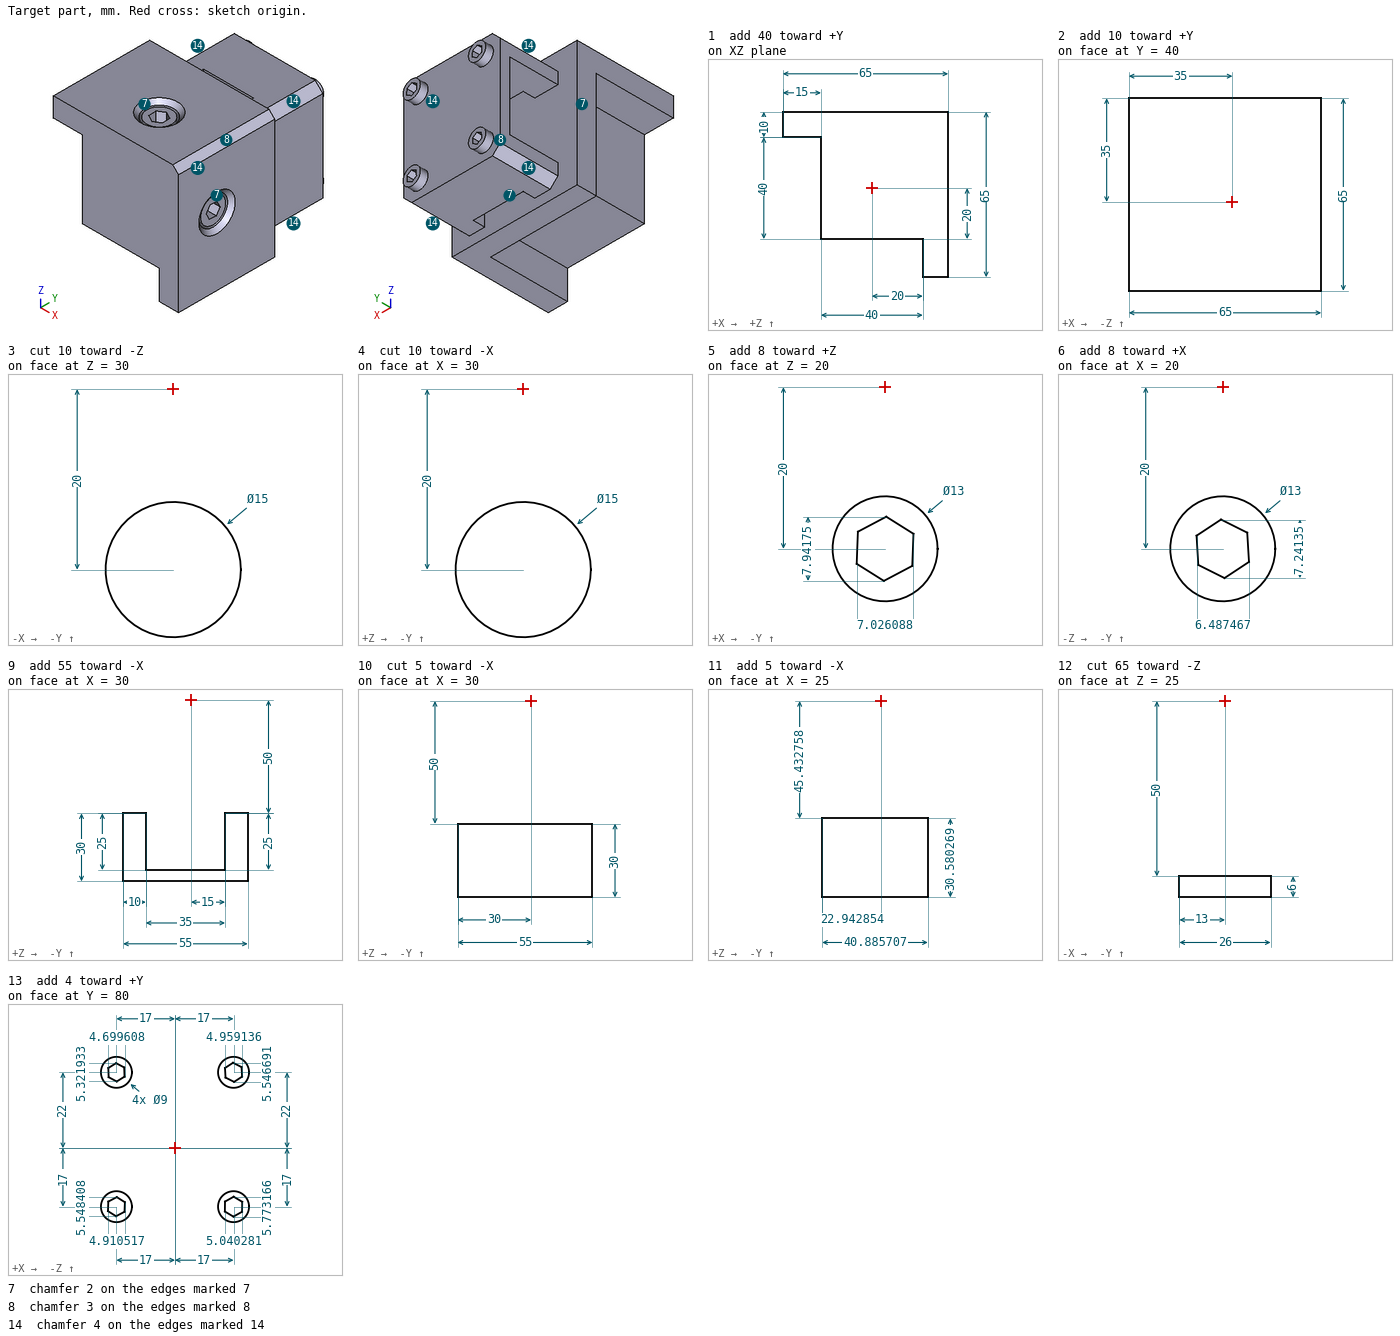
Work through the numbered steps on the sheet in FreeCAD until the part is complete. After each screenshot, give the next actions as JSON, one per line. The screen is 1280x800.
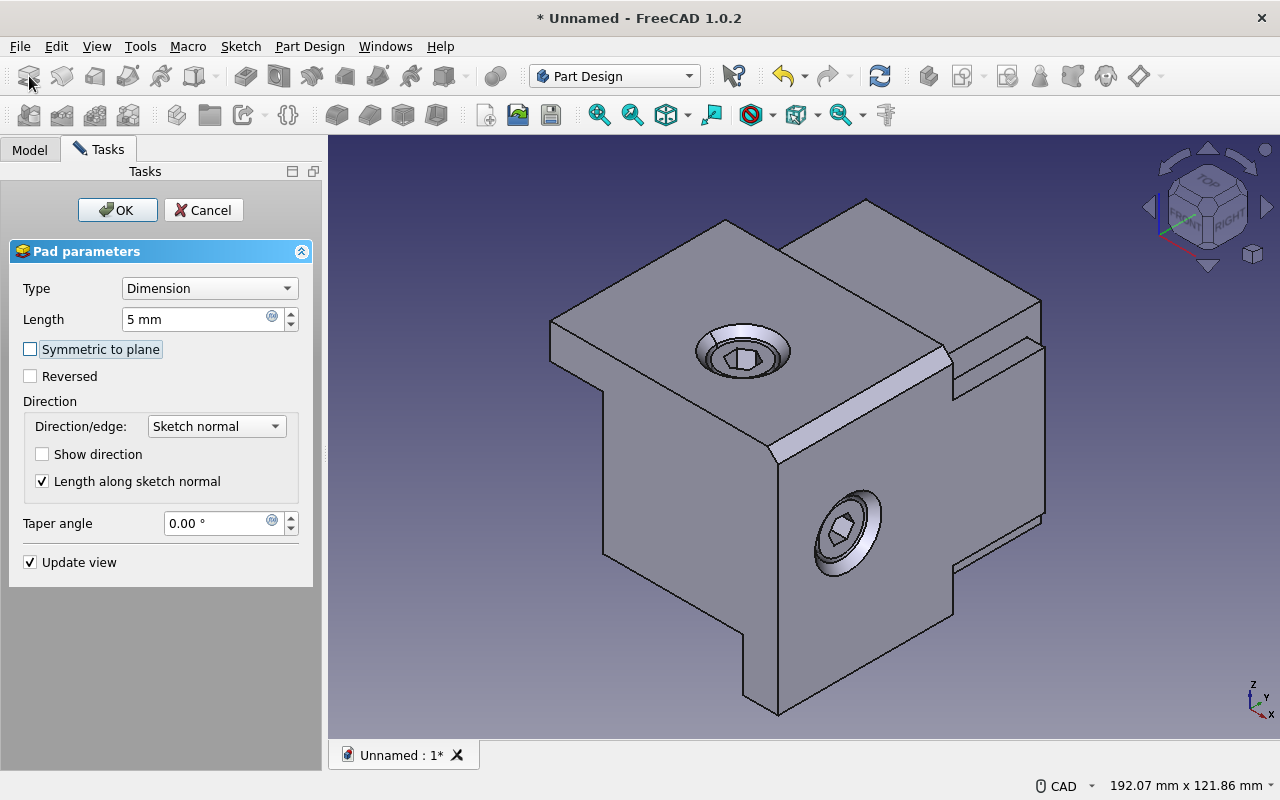
{"action": "left_click", "coordinate": [31, 376]}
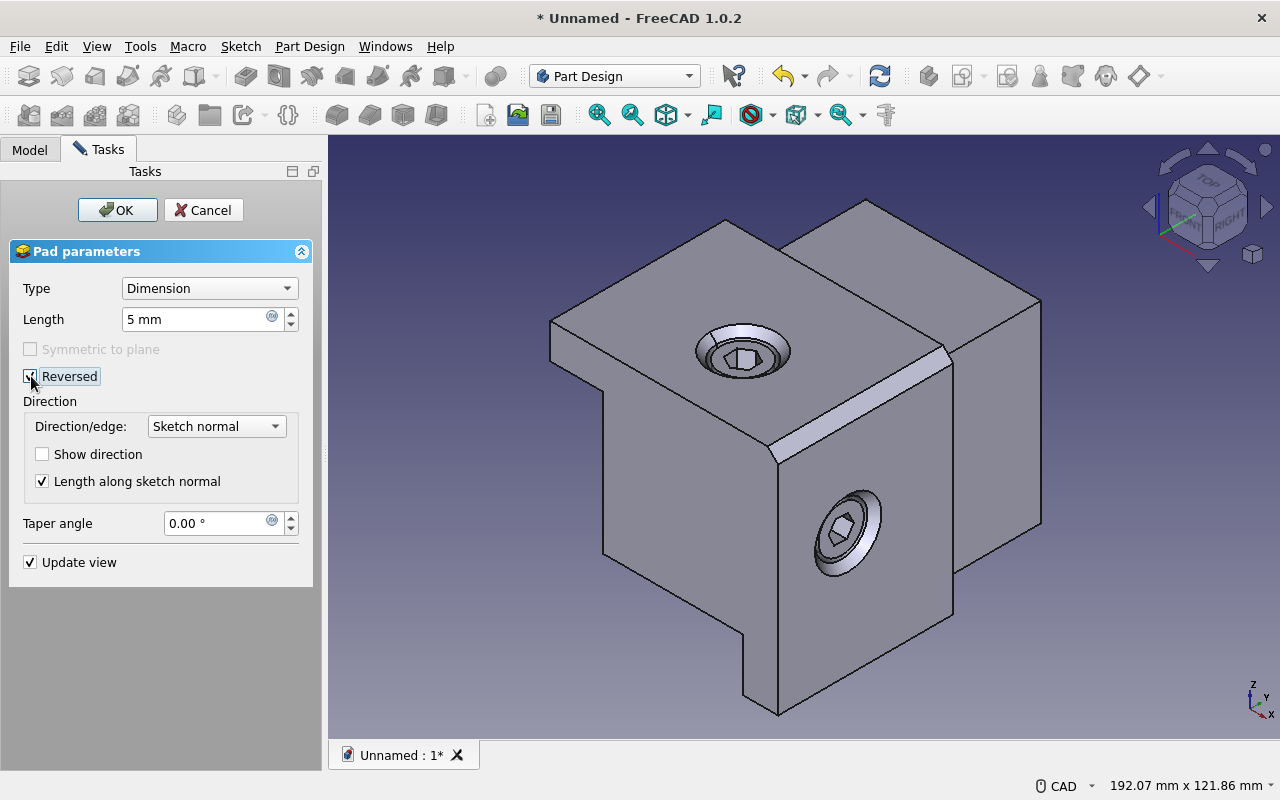
{"action": "left_click", "coordinate": [118, 210]}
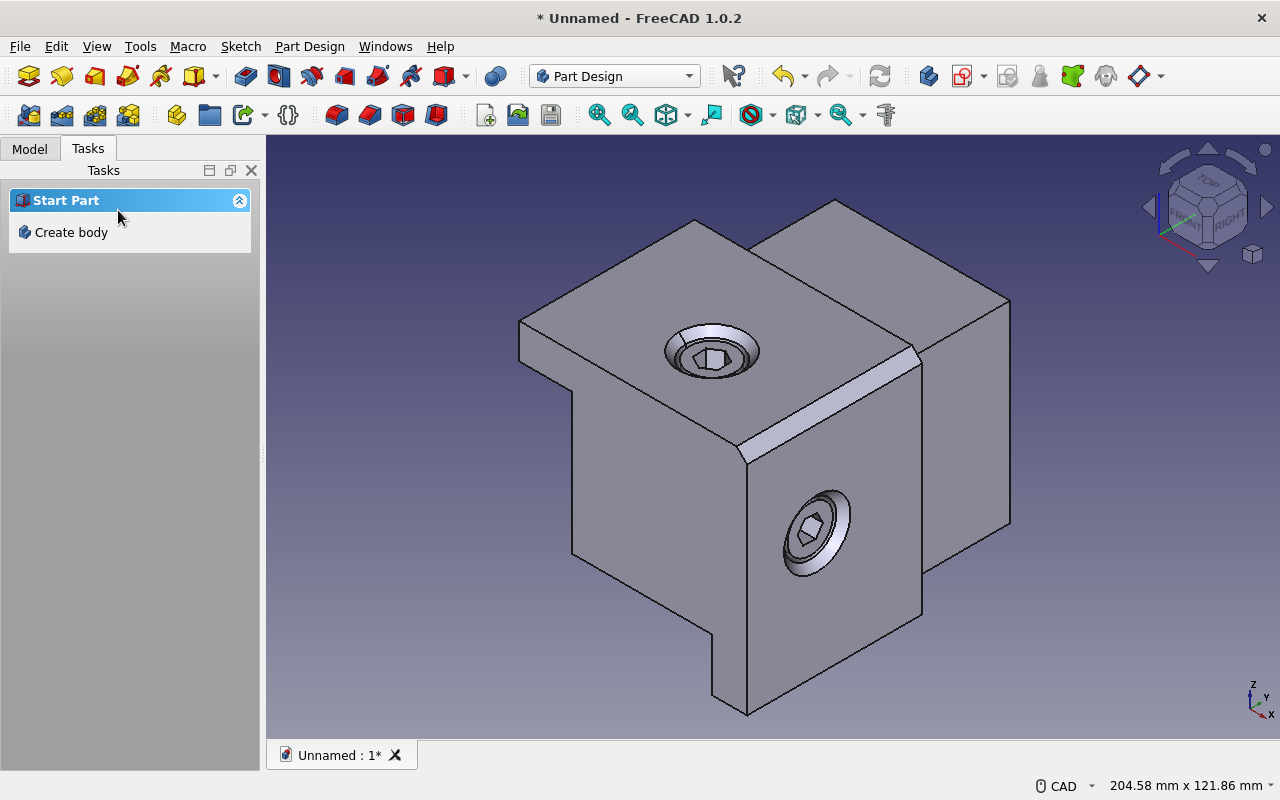
{"action": "left_click", "coordinate": [895, 294]}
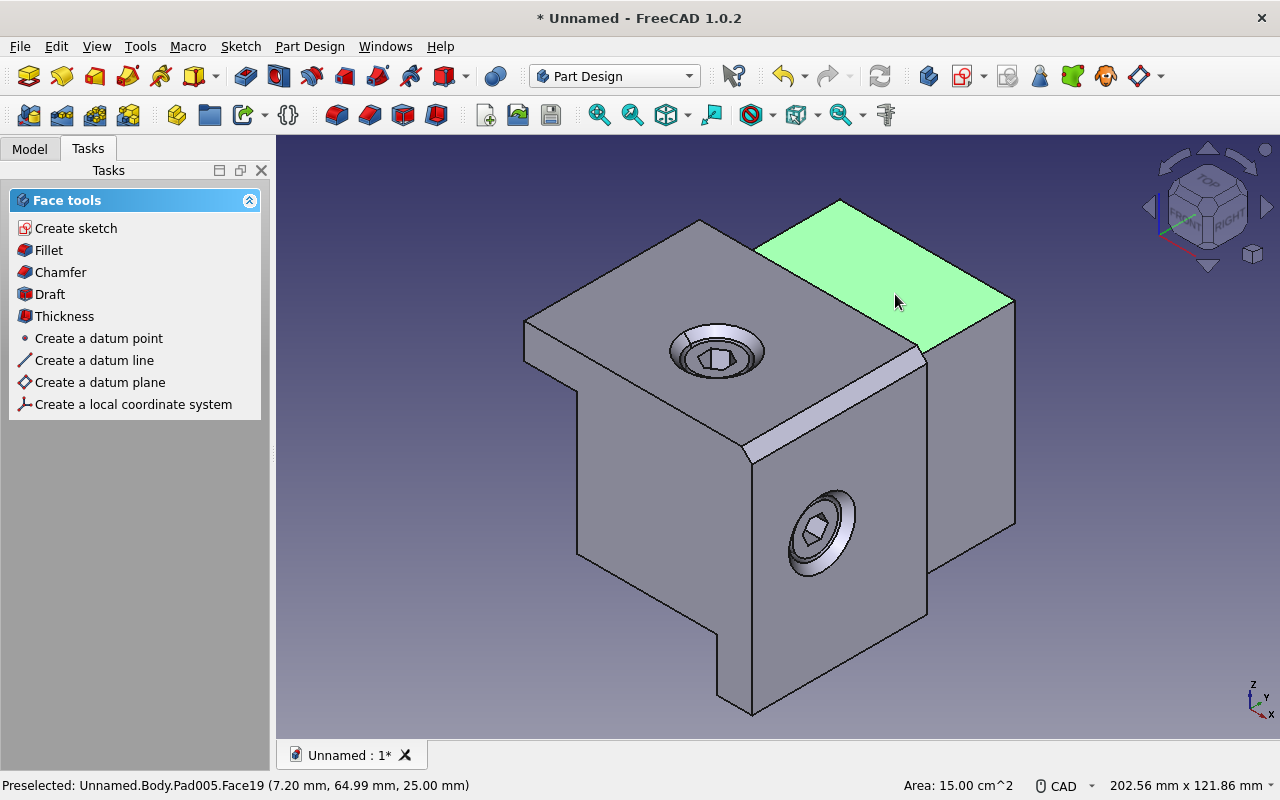
{"action": "left_click", "coordinate": [962, 76]}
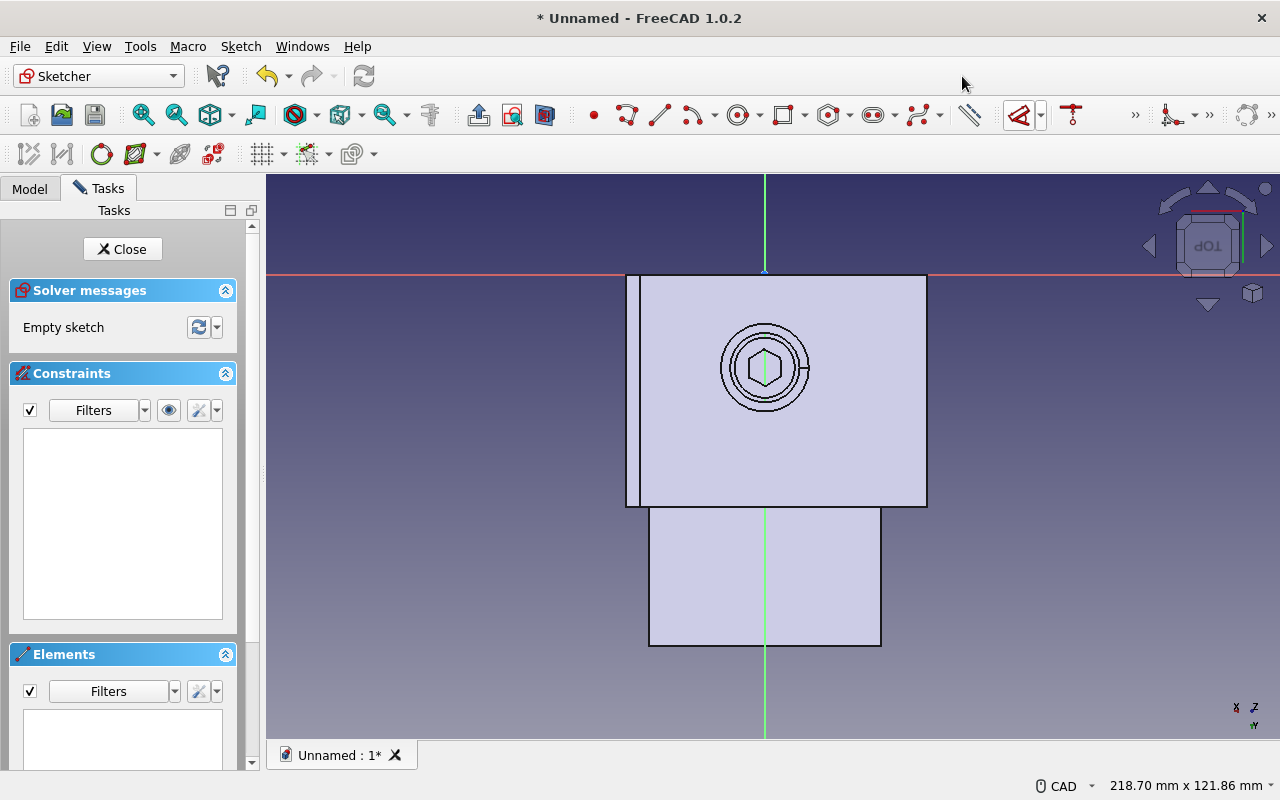
{"action": "scroll", "coordinate": [887, 300], "scroll_direction": "up", "scroll_amount": 2}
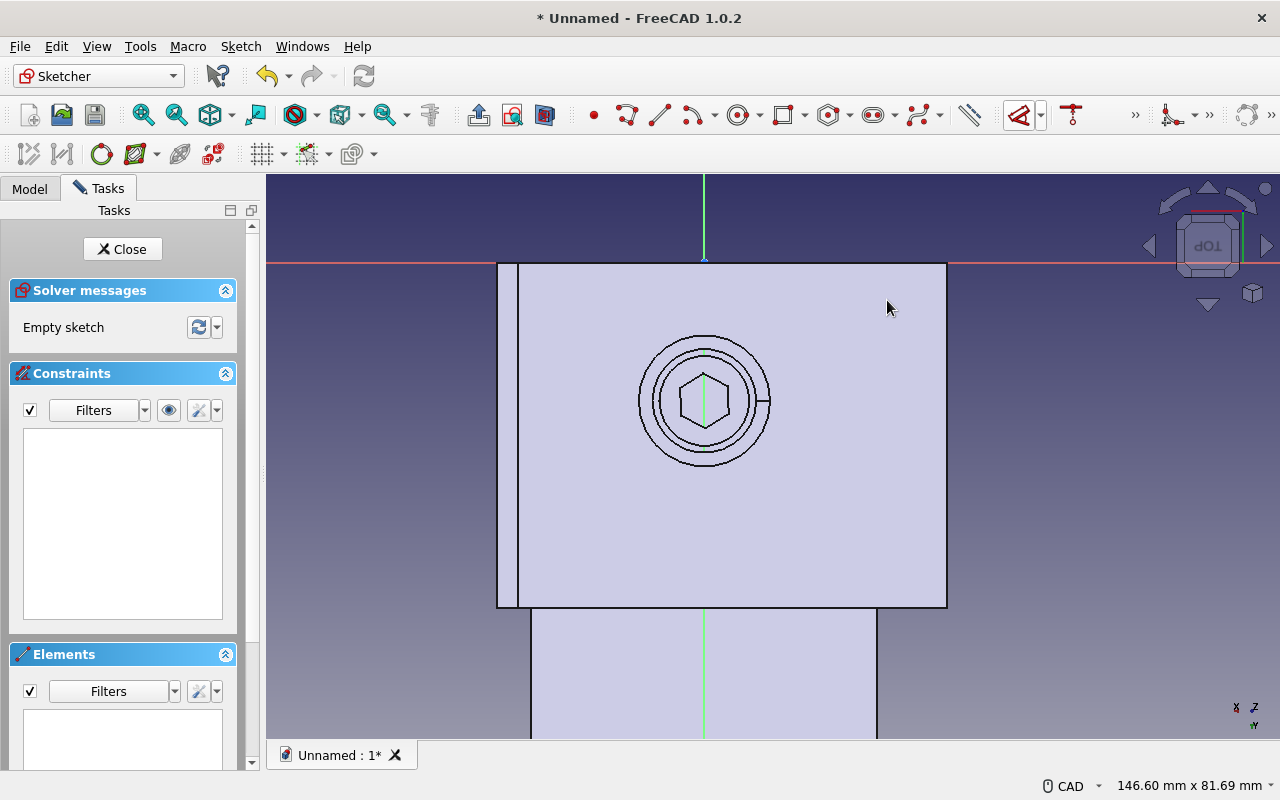
{"action": "left_click", "coordinate": [782, 116]}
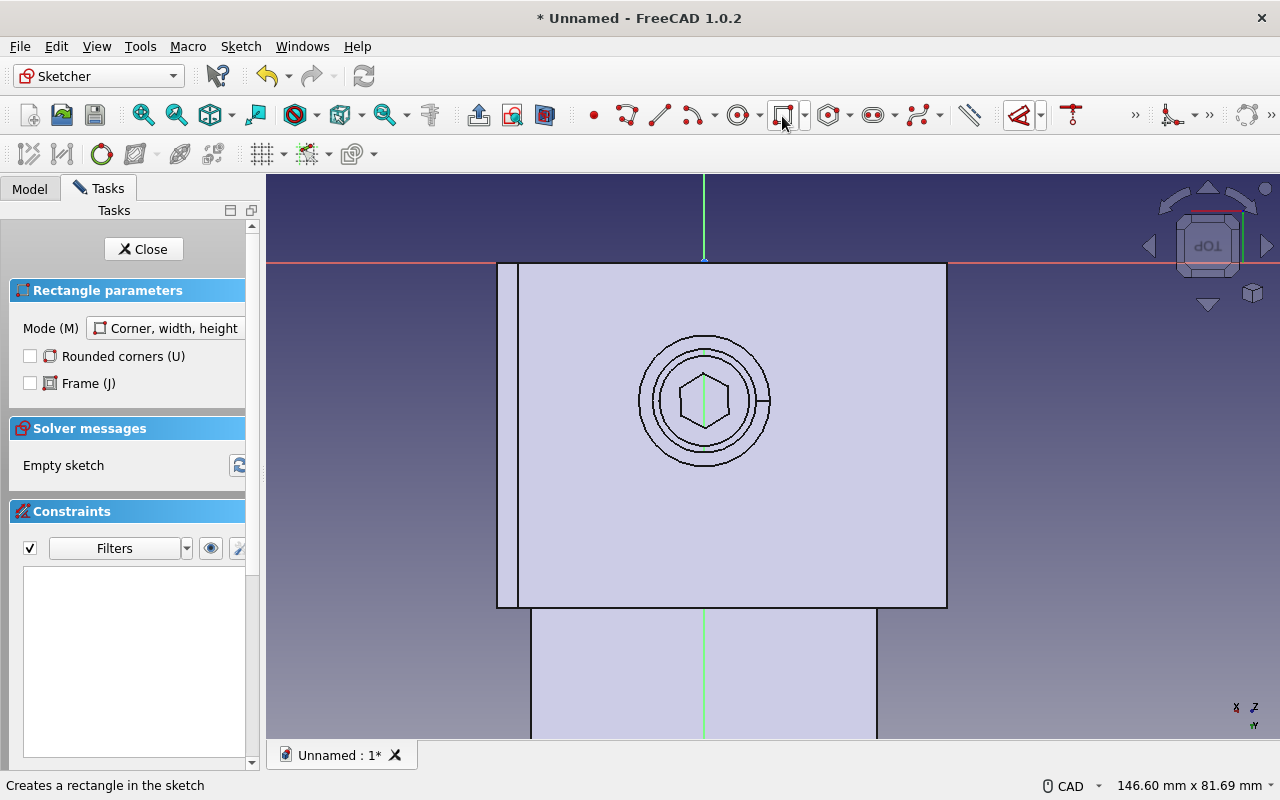
{"action": "left_click", "coordinate": [615, 608]}
{"action": "mouse_move", "coordinate": [794, 650]}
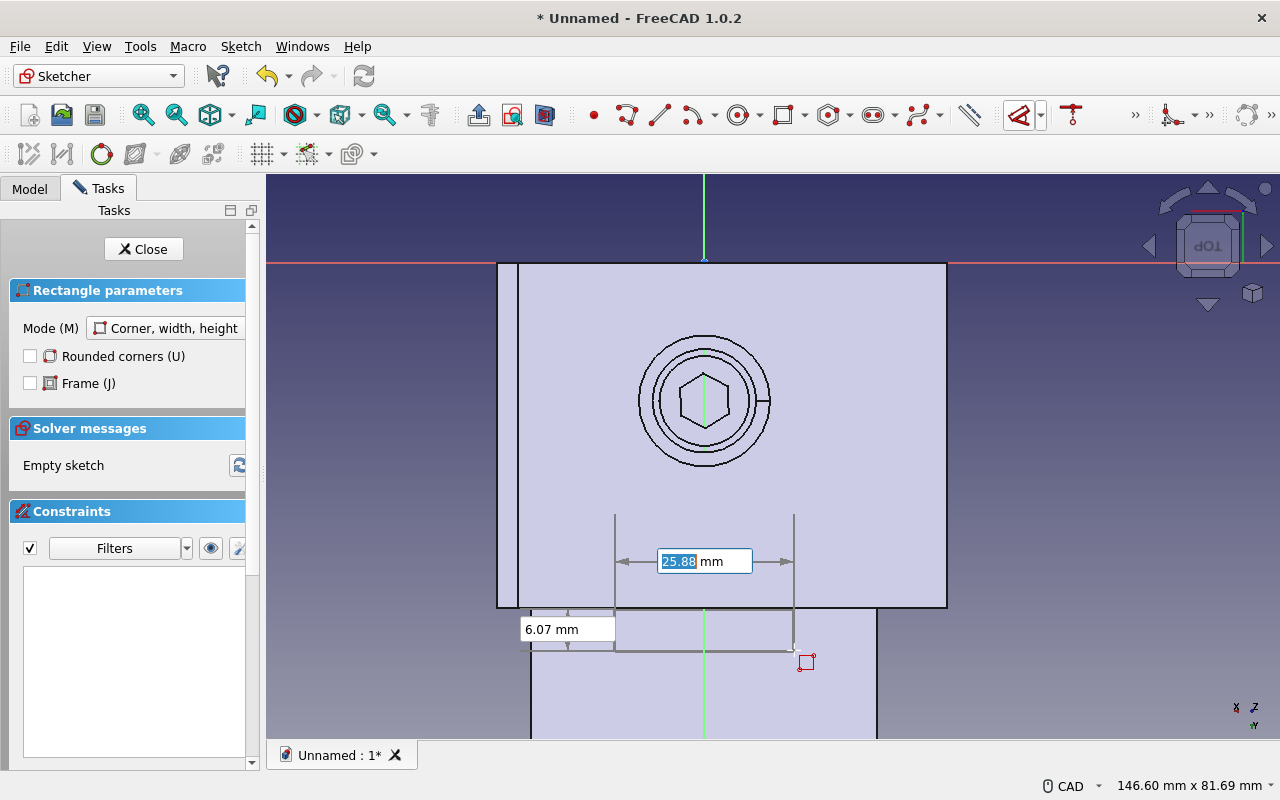
{"action": "type", "text": "26"}
{"action": "key", "text": "Tab"}
{"action": "type", "text": "6"}
{"action": "key", "text": "Return"}
{"action": "key", "text": "Escape"}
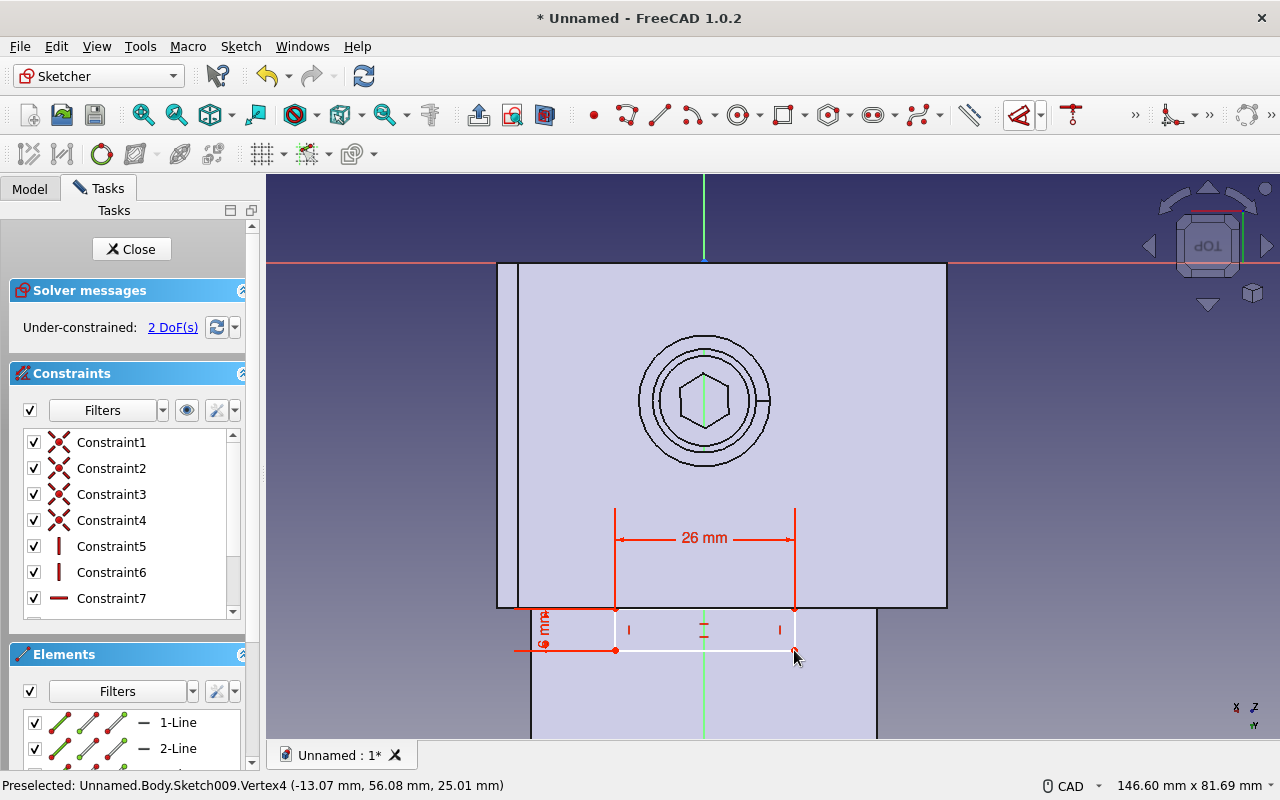
{"action": "left_click", "coordinate": [615, 609]}